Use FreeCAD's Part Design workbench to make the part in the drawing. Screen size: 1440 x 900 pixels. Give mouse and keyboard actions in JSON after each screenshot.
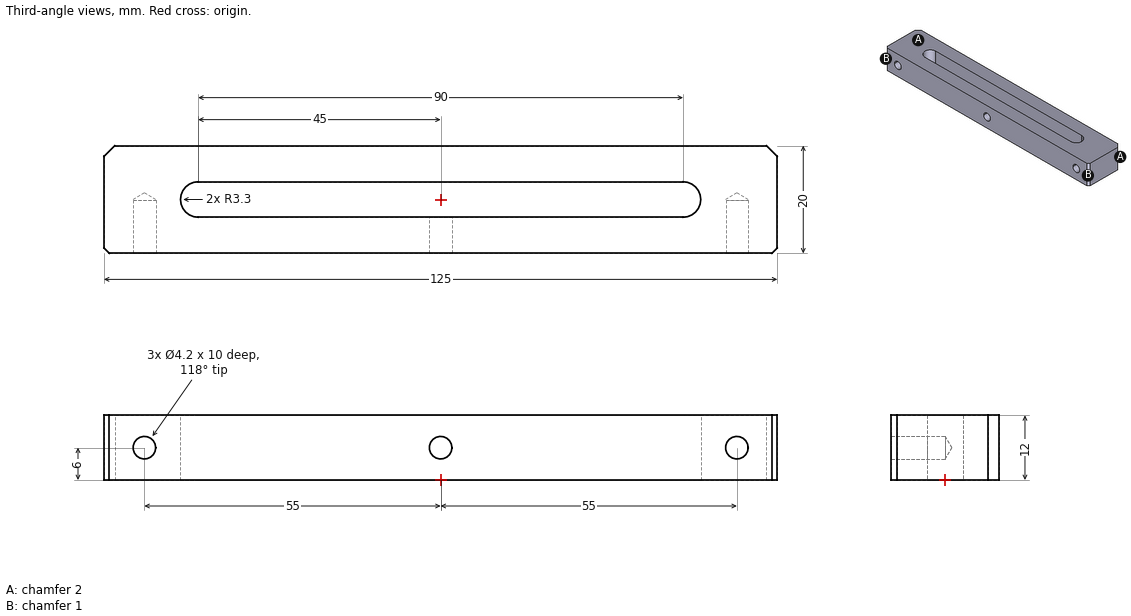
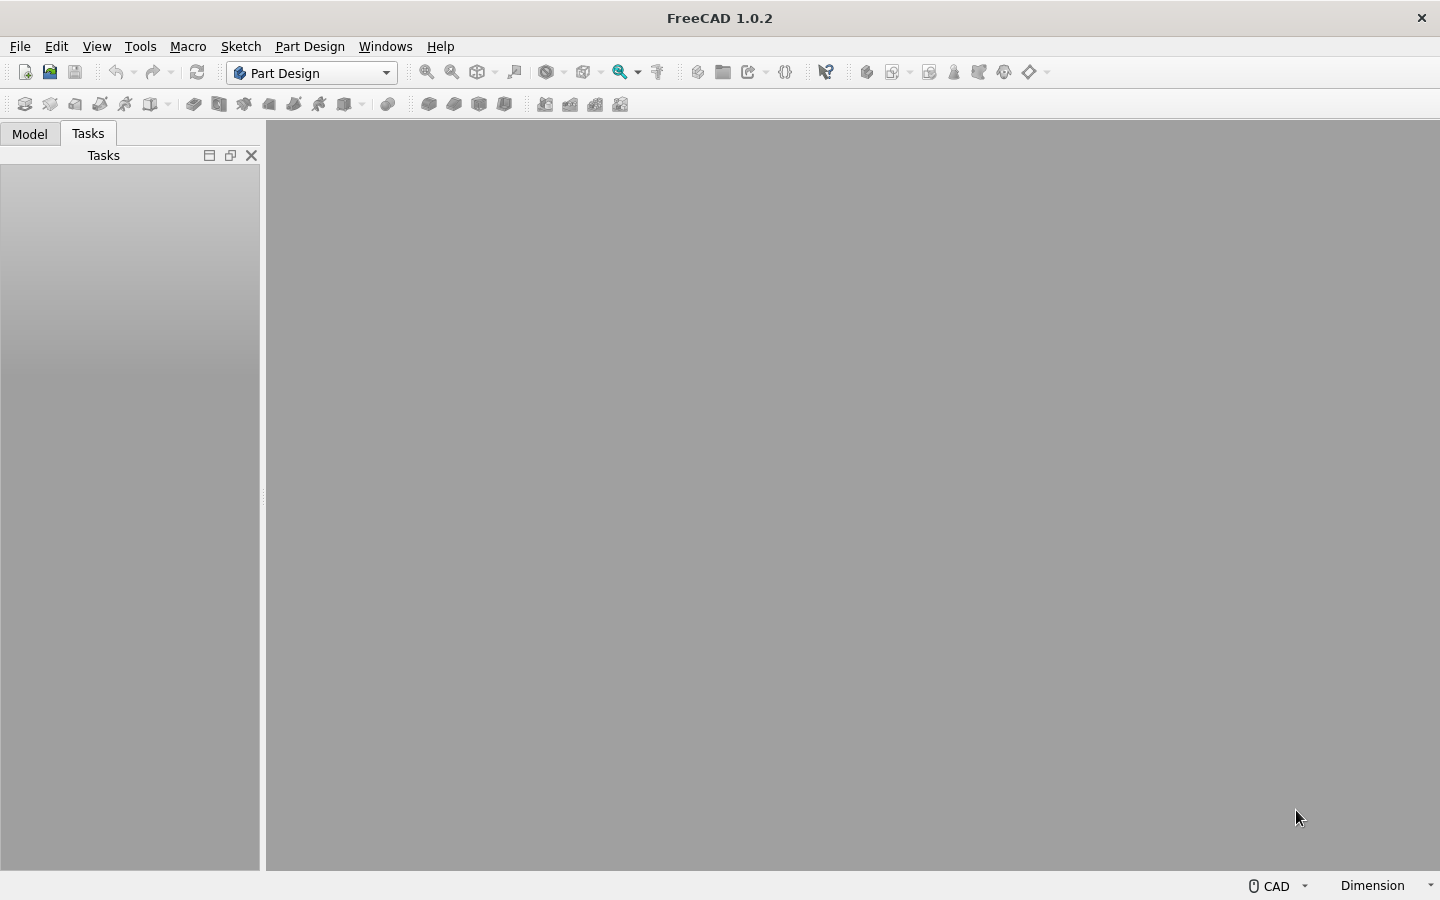
{"action": "left_click", "coordinate": [25, 72]}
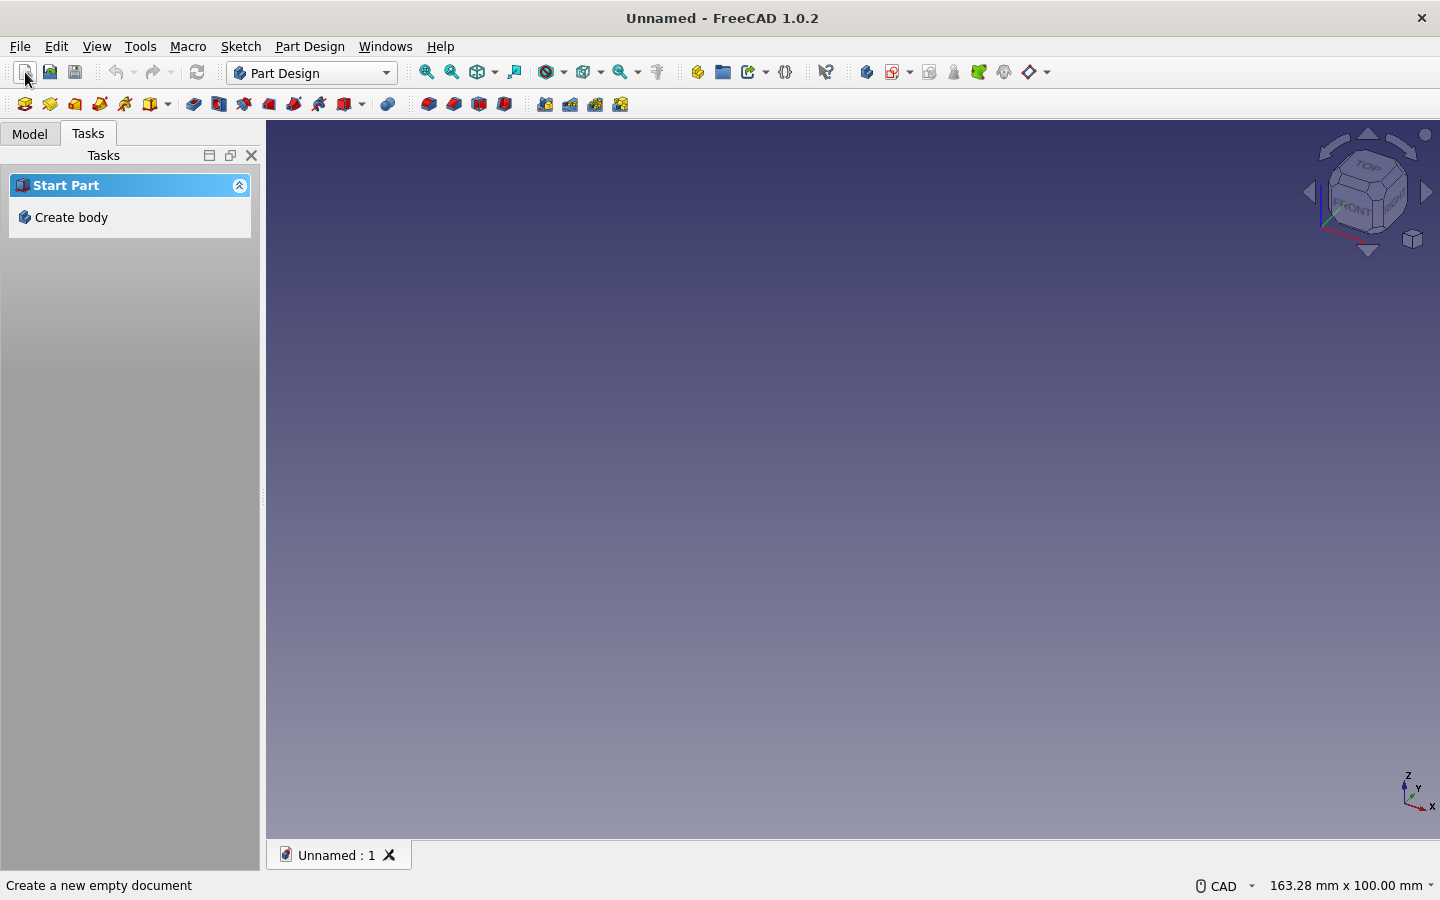
{"action": "left_click", "coordinate": [892, 72]}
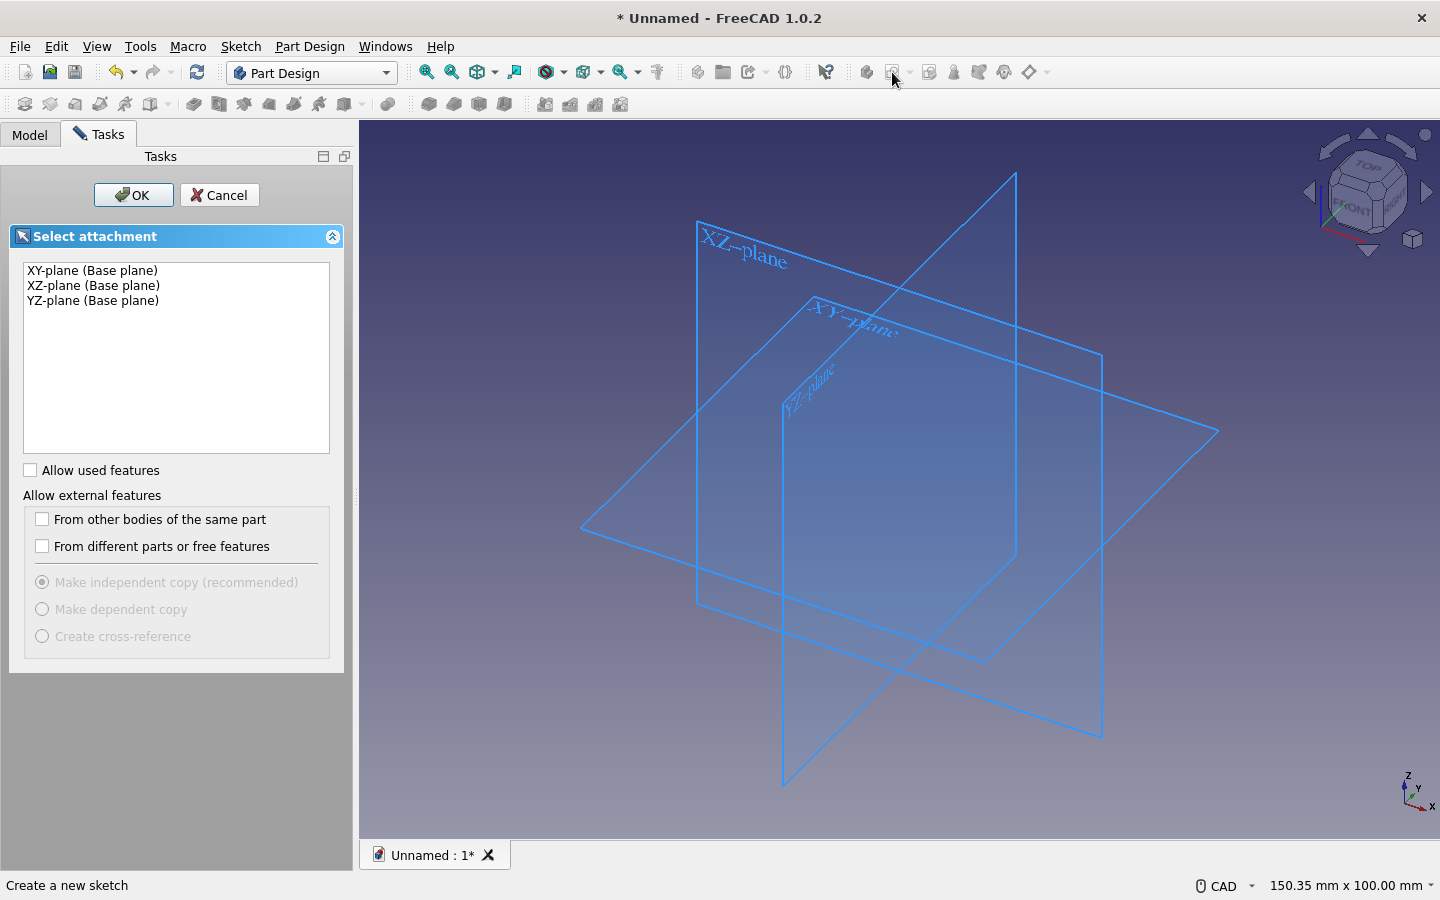
{"action": "left_click", "coordinate": [84, 270]}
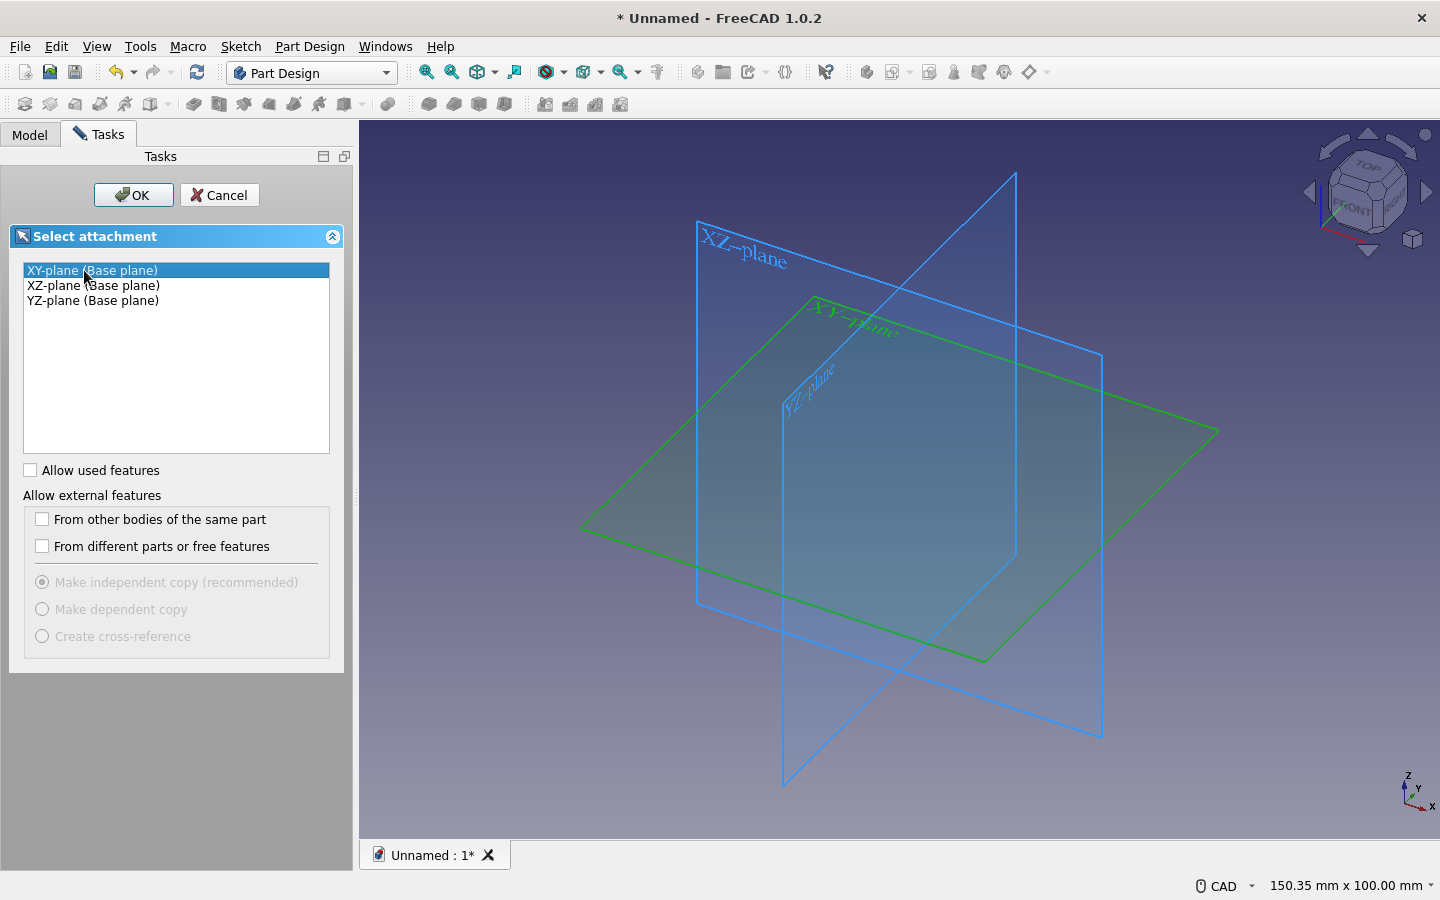
{"action": "left_click", "coordinate": [134, 195]}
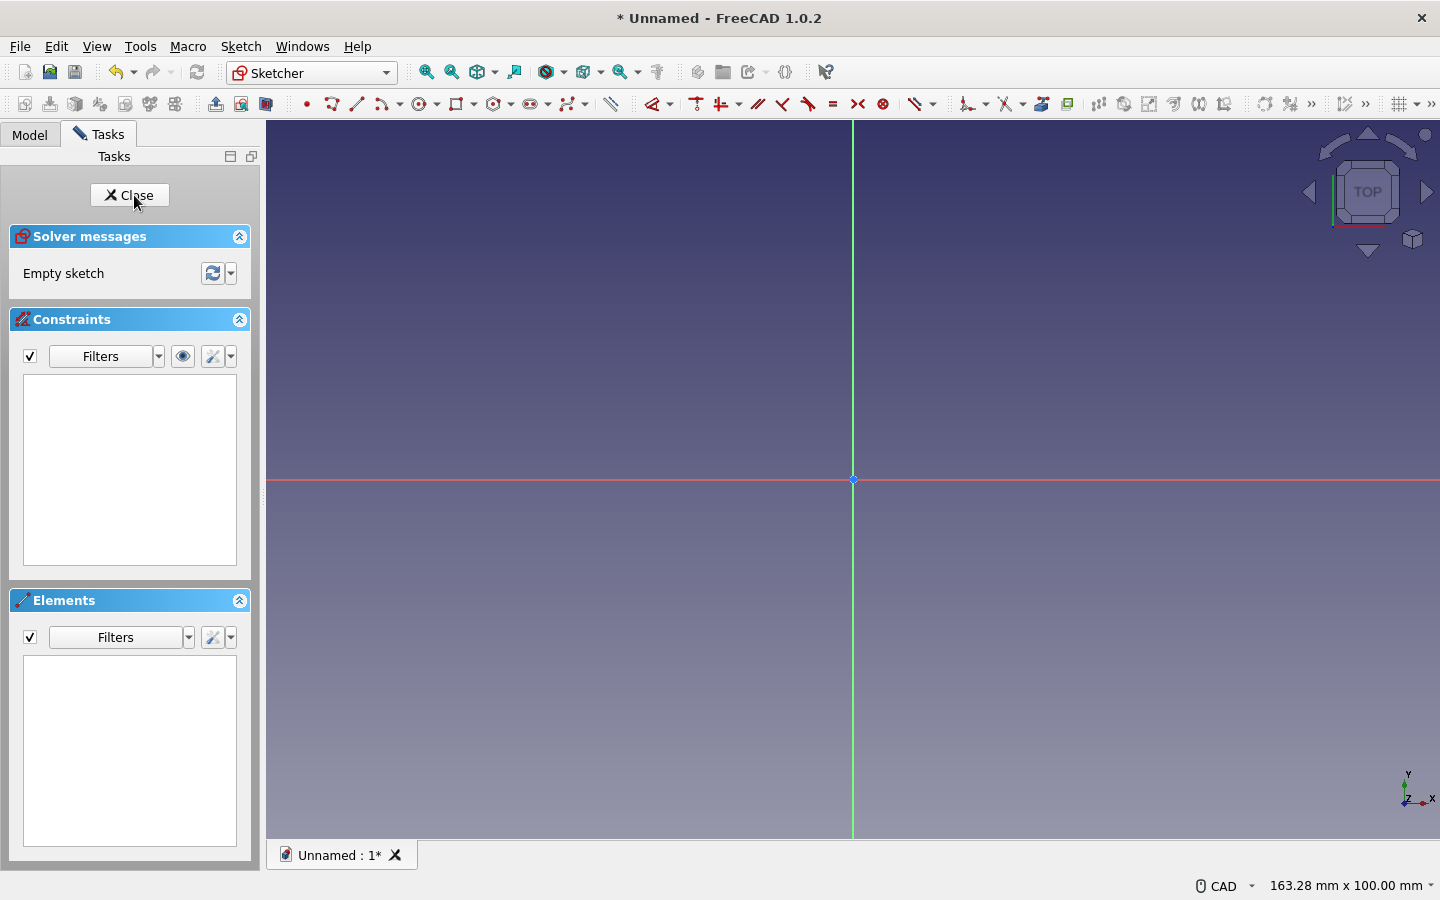
{"action": "scroll", "coordinate": [475, 480], "scroll_direction": "down", "scroll_amount": 1}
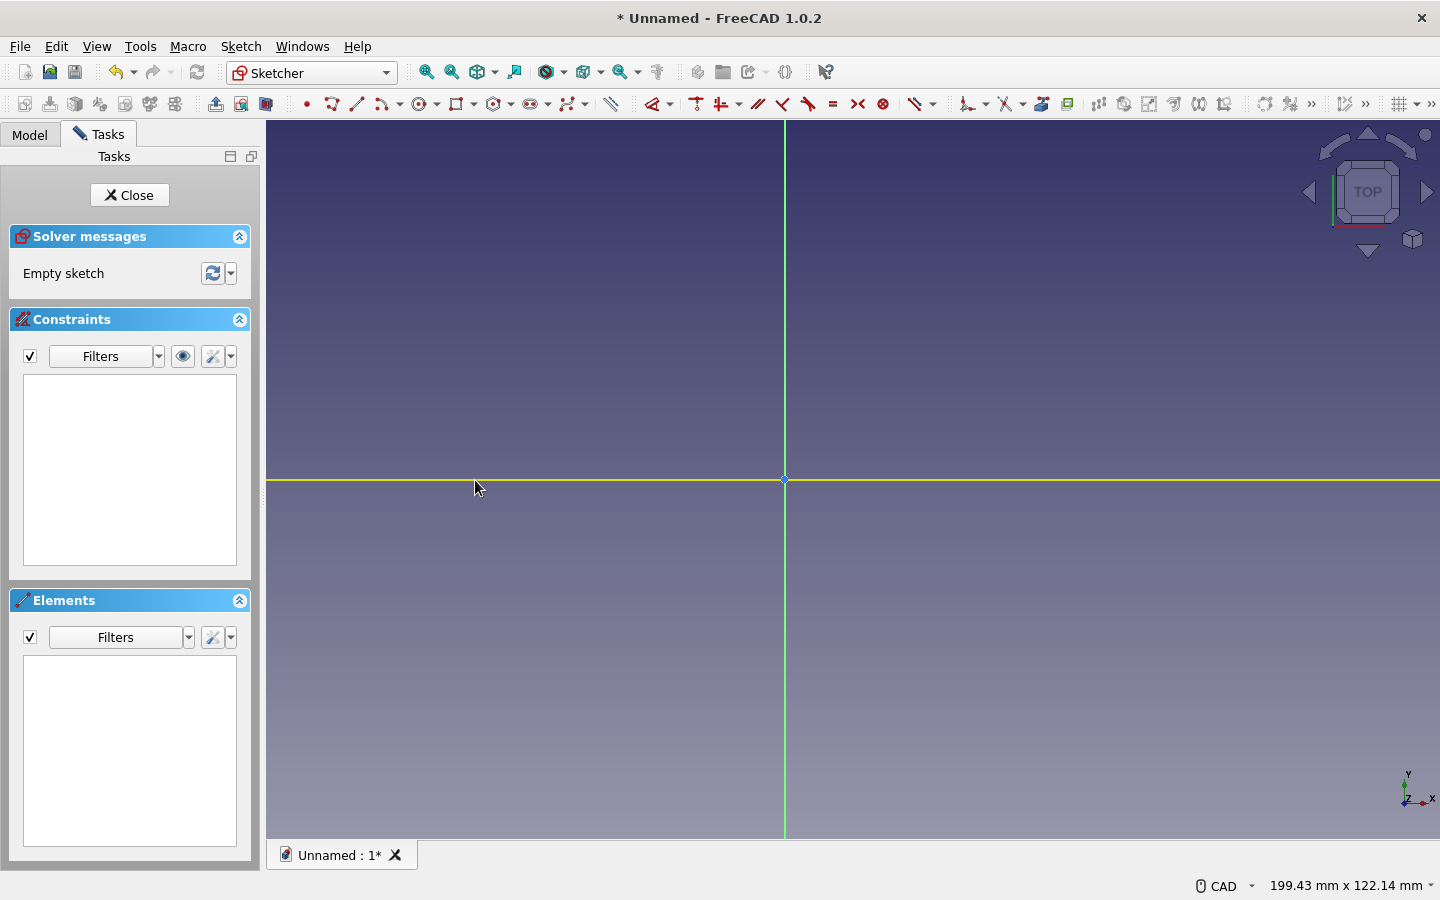
{"action": "key", "text": "g v"}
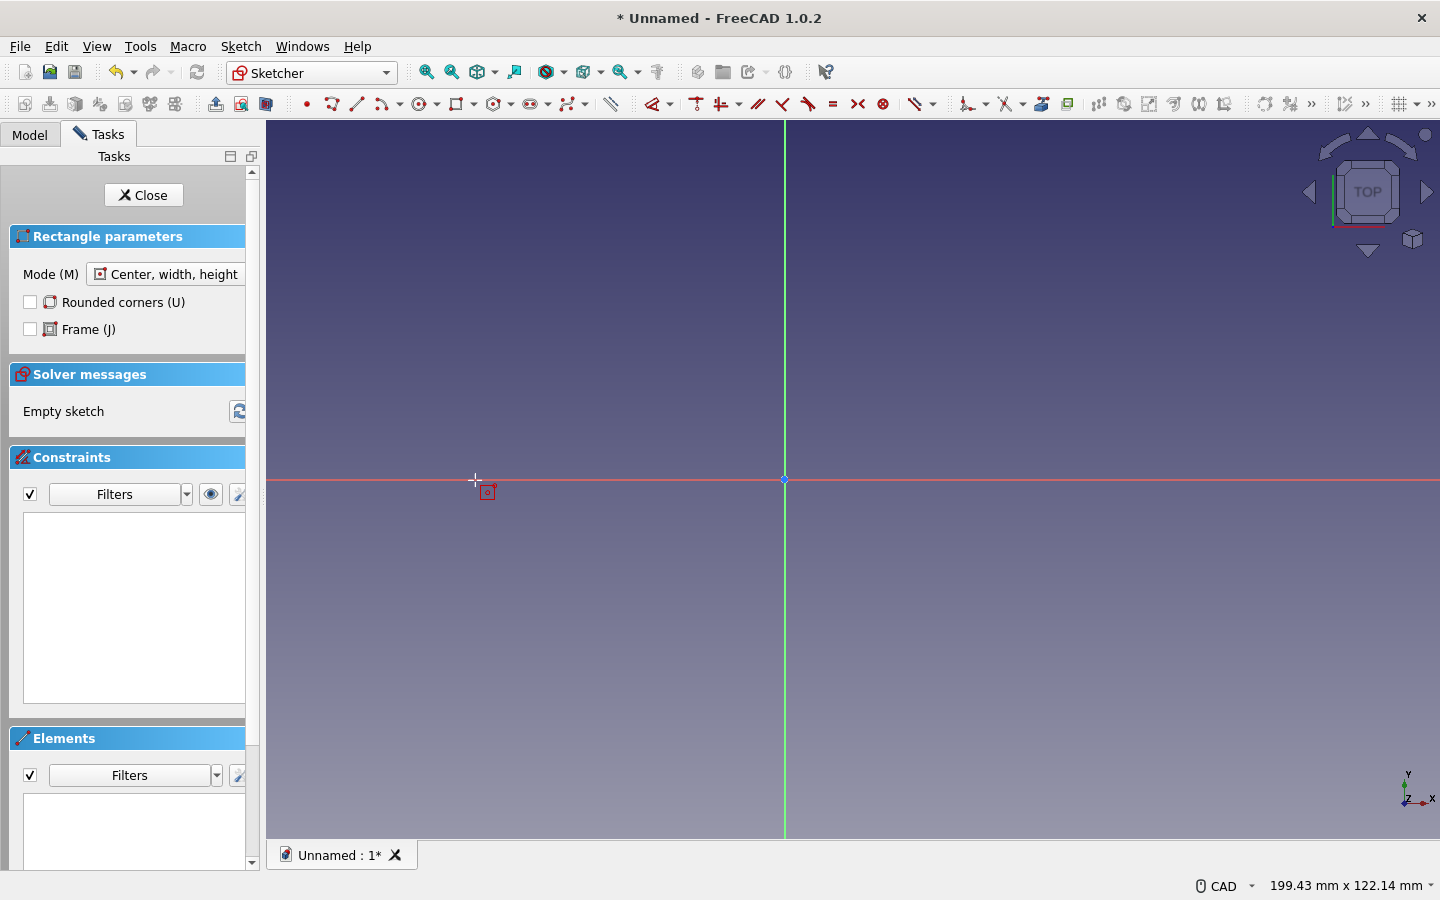
{"action": "left_click", "coordinate": [785, 480]}
{"action": "mouse_move", "coordinate": [1152, 421]}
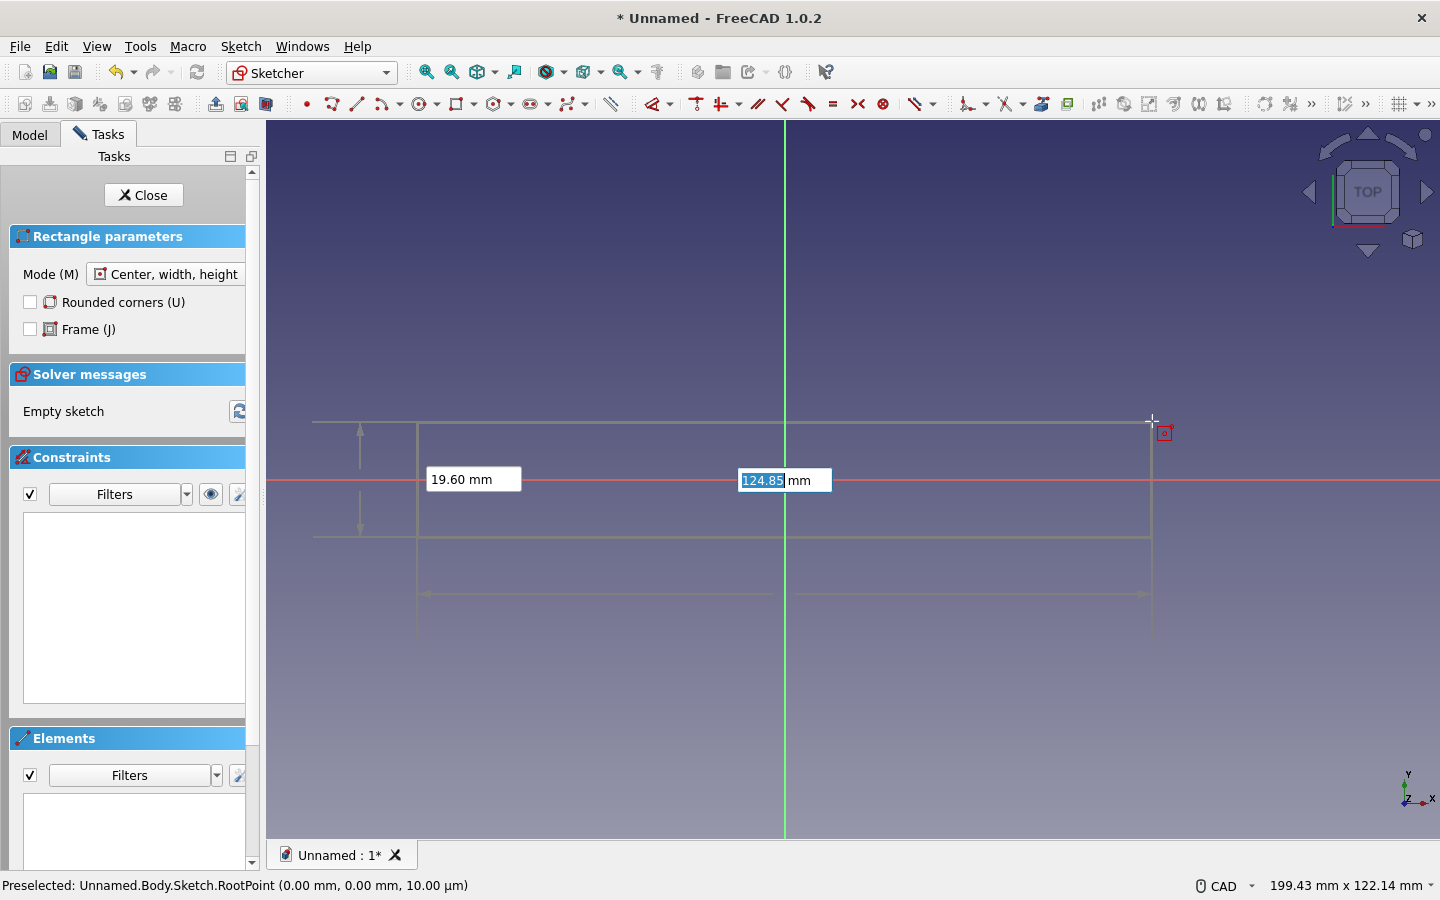
{"action": "type", "text": "125"}
{"action": "key", "text": "Tab"}
{"action": "type", "text": "20"}
{"action": "key", "text": "Return"}
{"action": "key", "text": "Escape"}